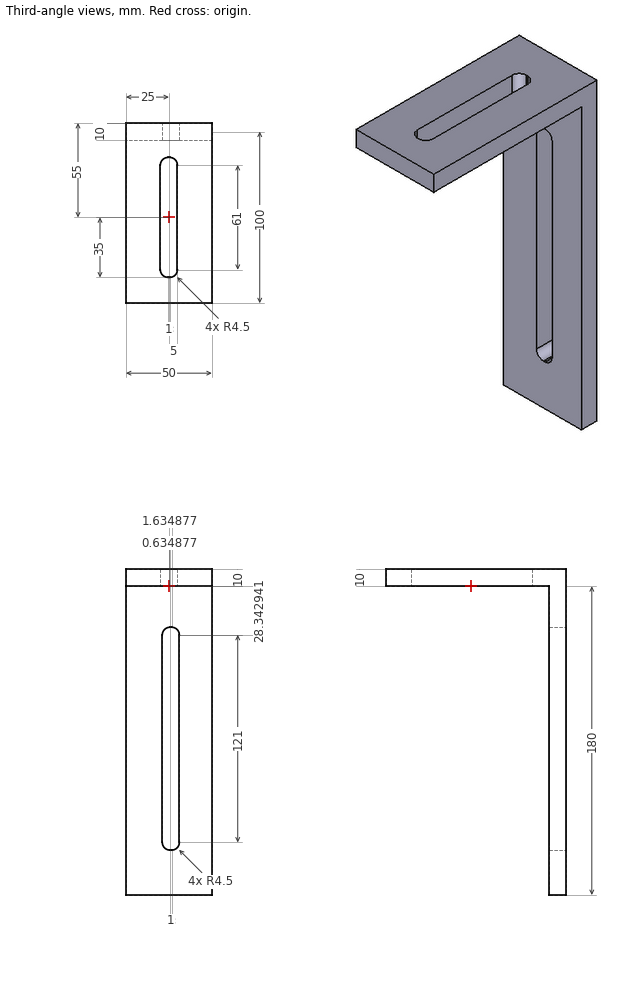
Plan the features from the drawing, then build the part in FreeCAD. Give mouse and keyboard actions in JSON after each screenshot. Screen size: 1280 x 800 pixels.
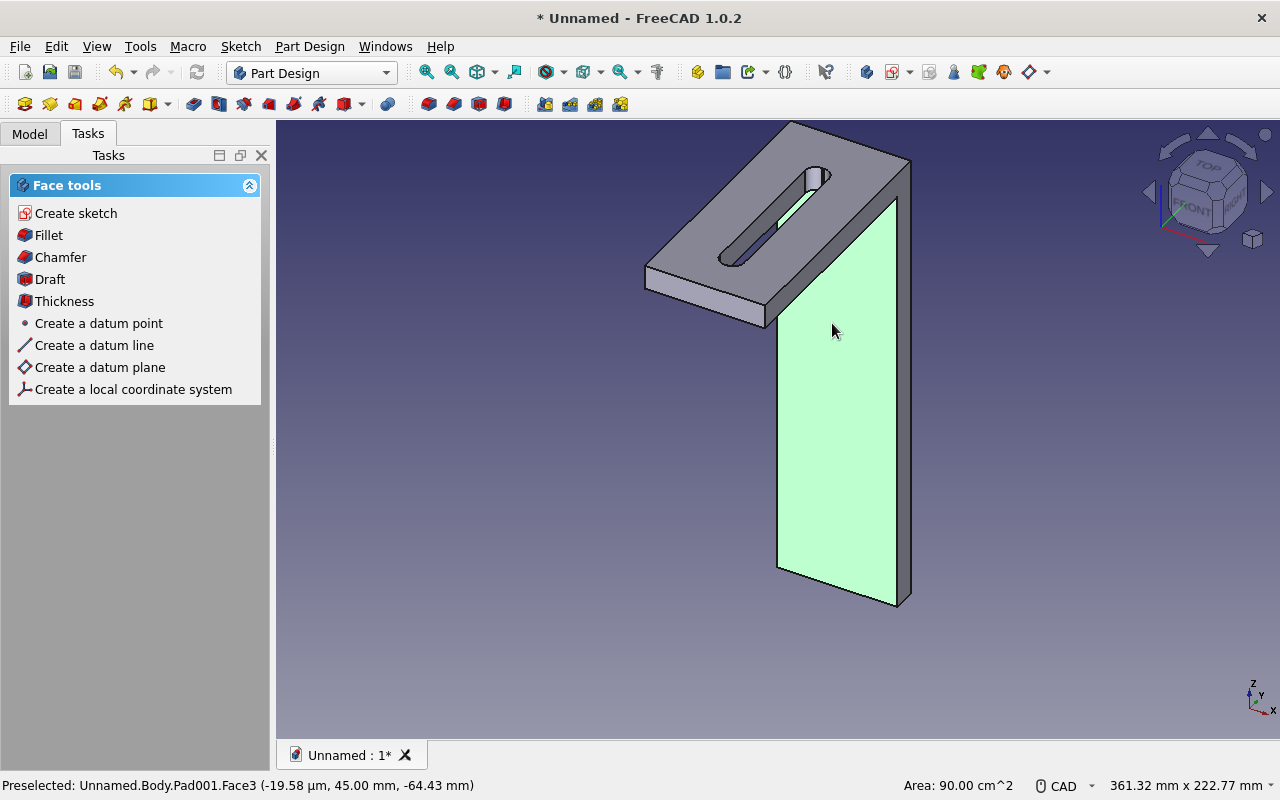
{"action": "left_click", "coordinate": [892, 72]}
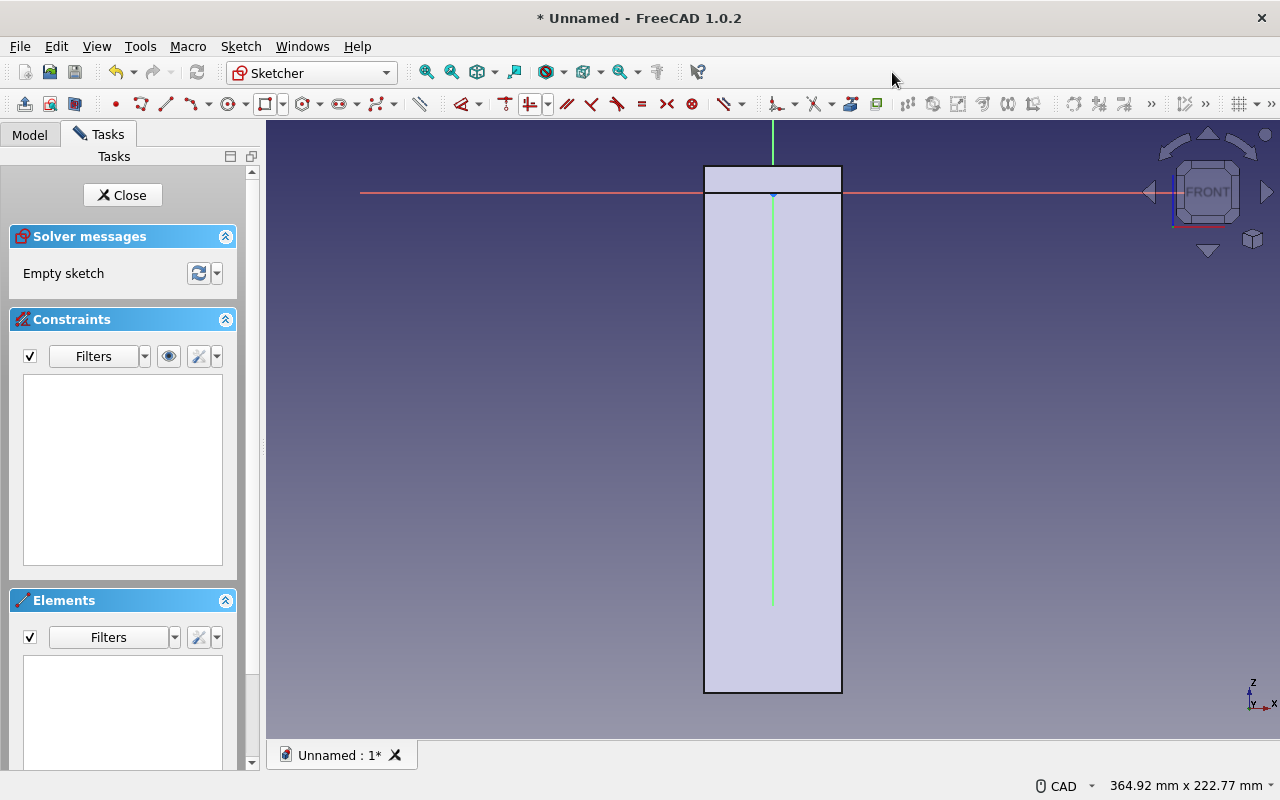
{"action": "left_click", "coordinate": [166, 104]}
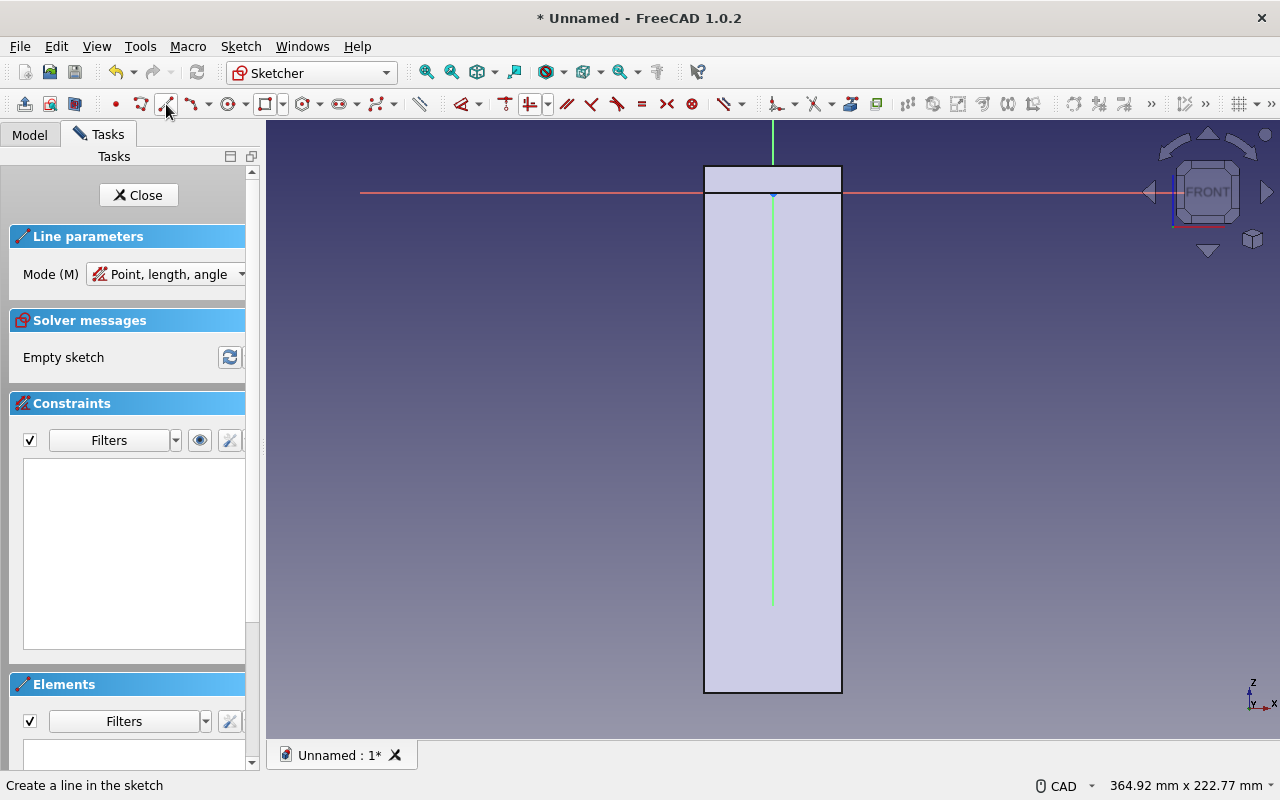
{"action": "scroll", "coordinate": [775, 621], "scroll_direction": "up", "scroll_amount": 11}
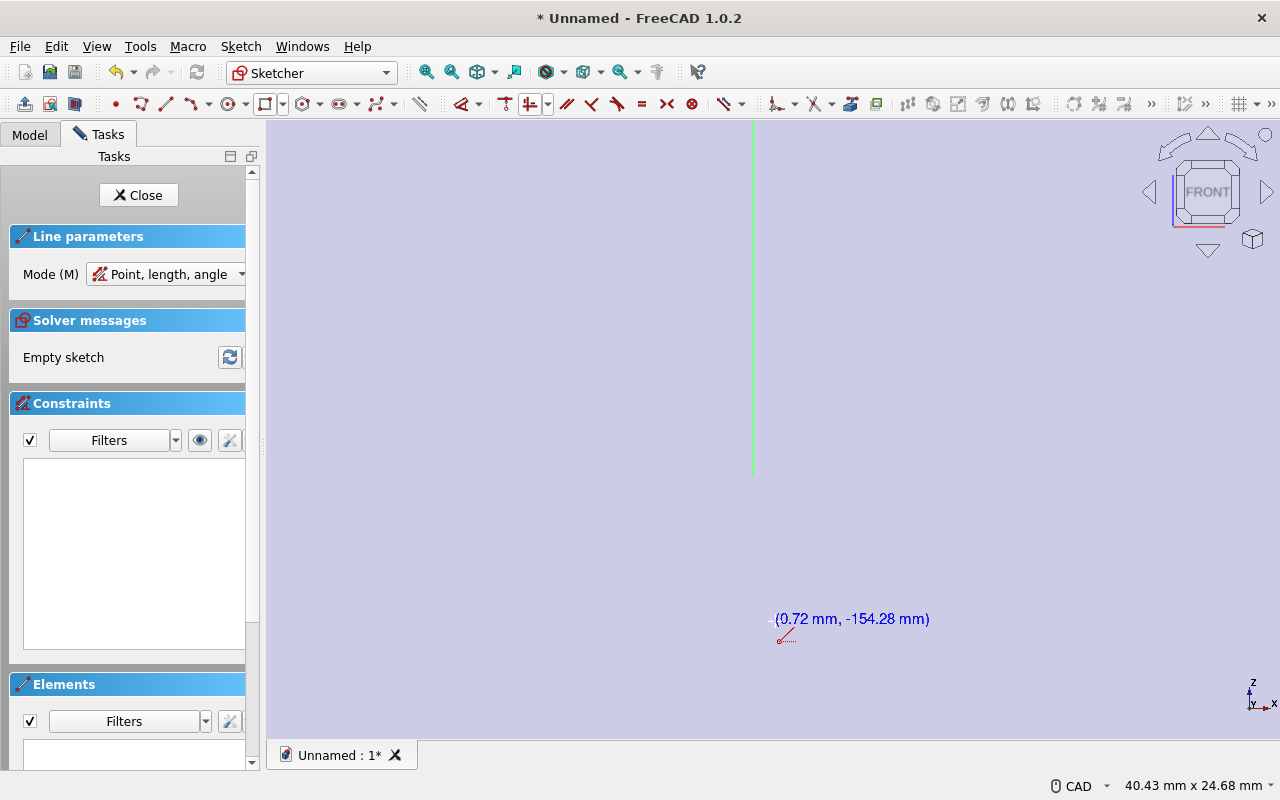
{"action": "left_click", "coordinate": [769, 613]}
{"action": "left_click", "coordinate": [794, 613]}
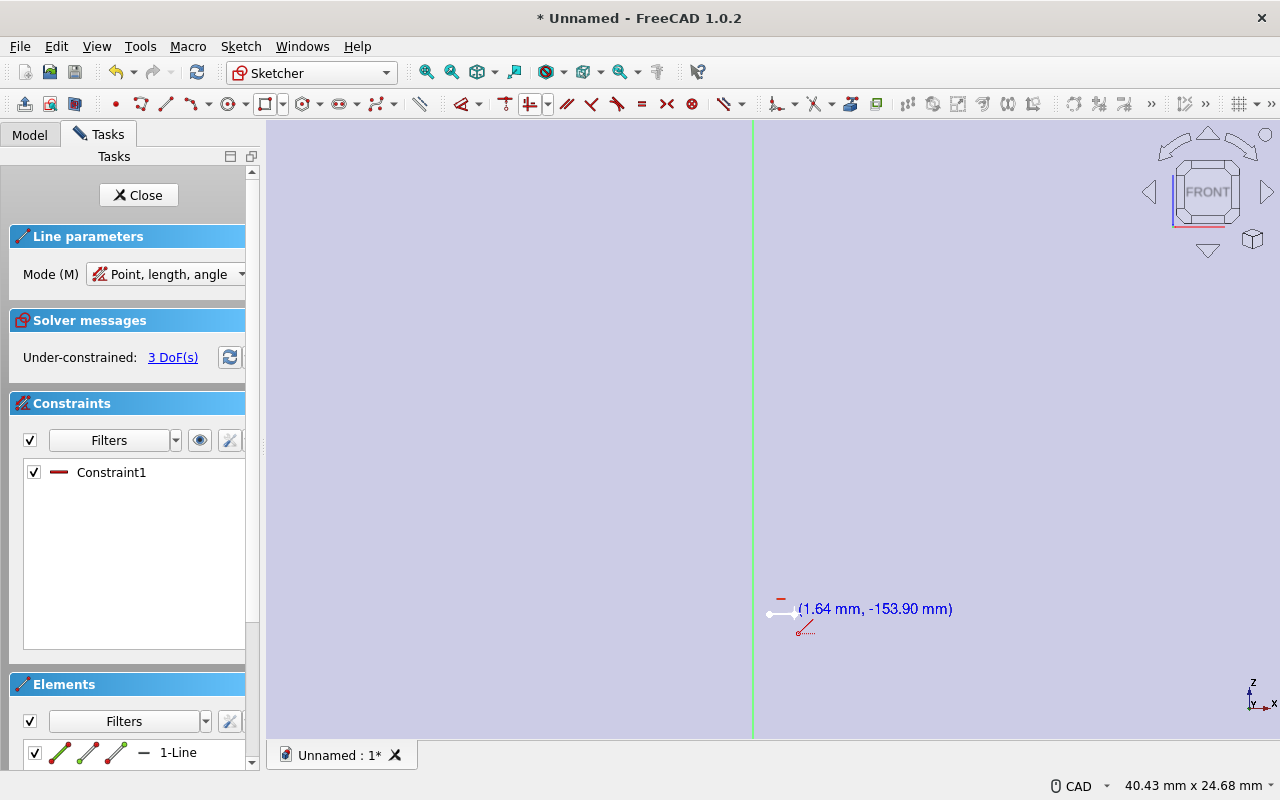
{"action": "scroll", "coordinate": [695, 647], "scroll_direction": "down", "scroll_amount": 11}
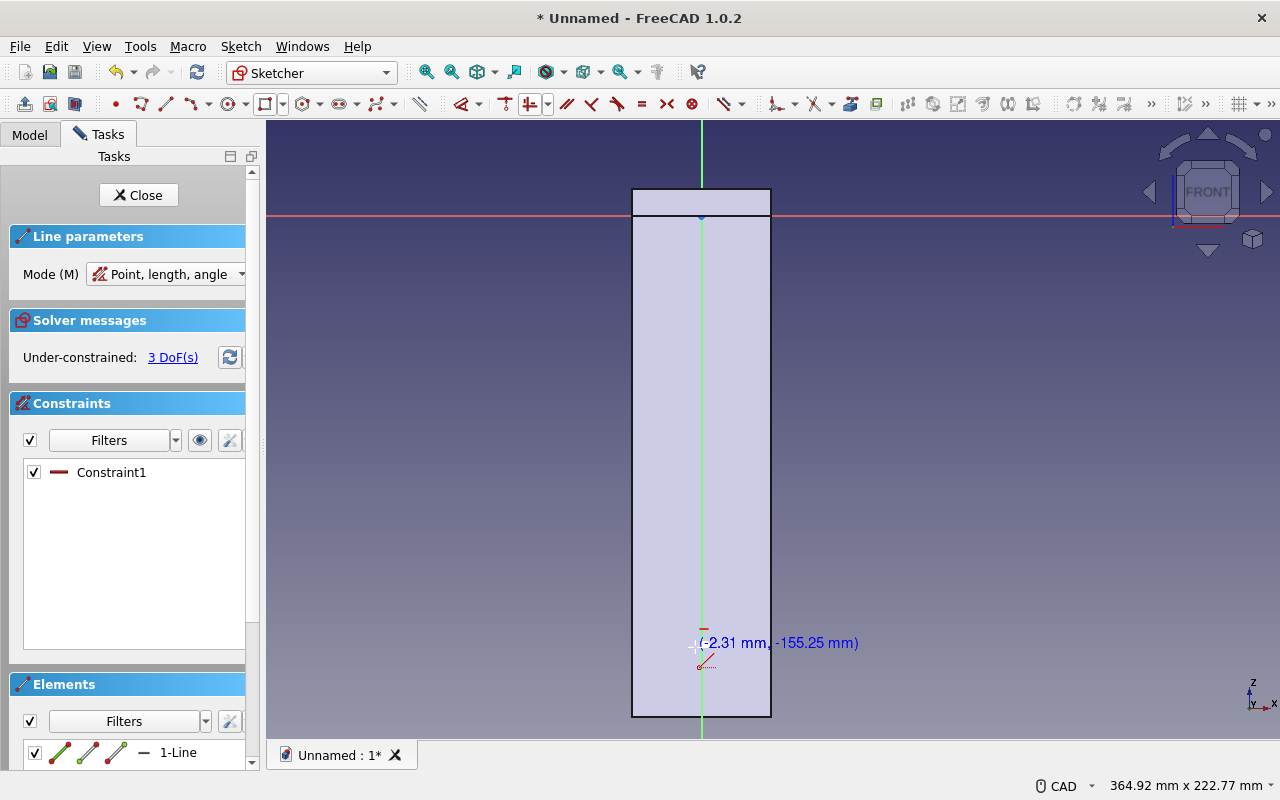
{"action": "left_click", "coordinate": [719, 631]}
{"action": "left_click", "coordinate": [719, 295]}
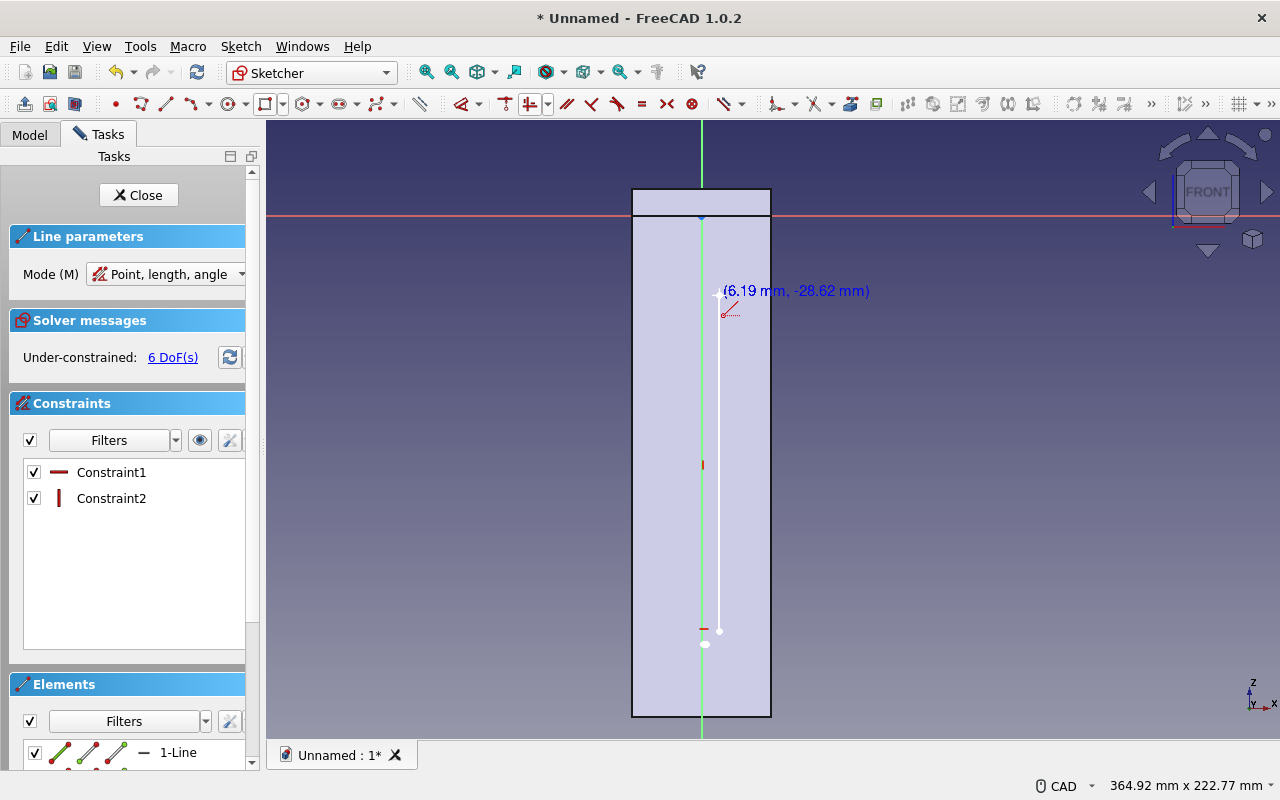
{"action": "scroll", "coordinate": [706, 283], "scroll_direction": "up", "scroll_amount": 7}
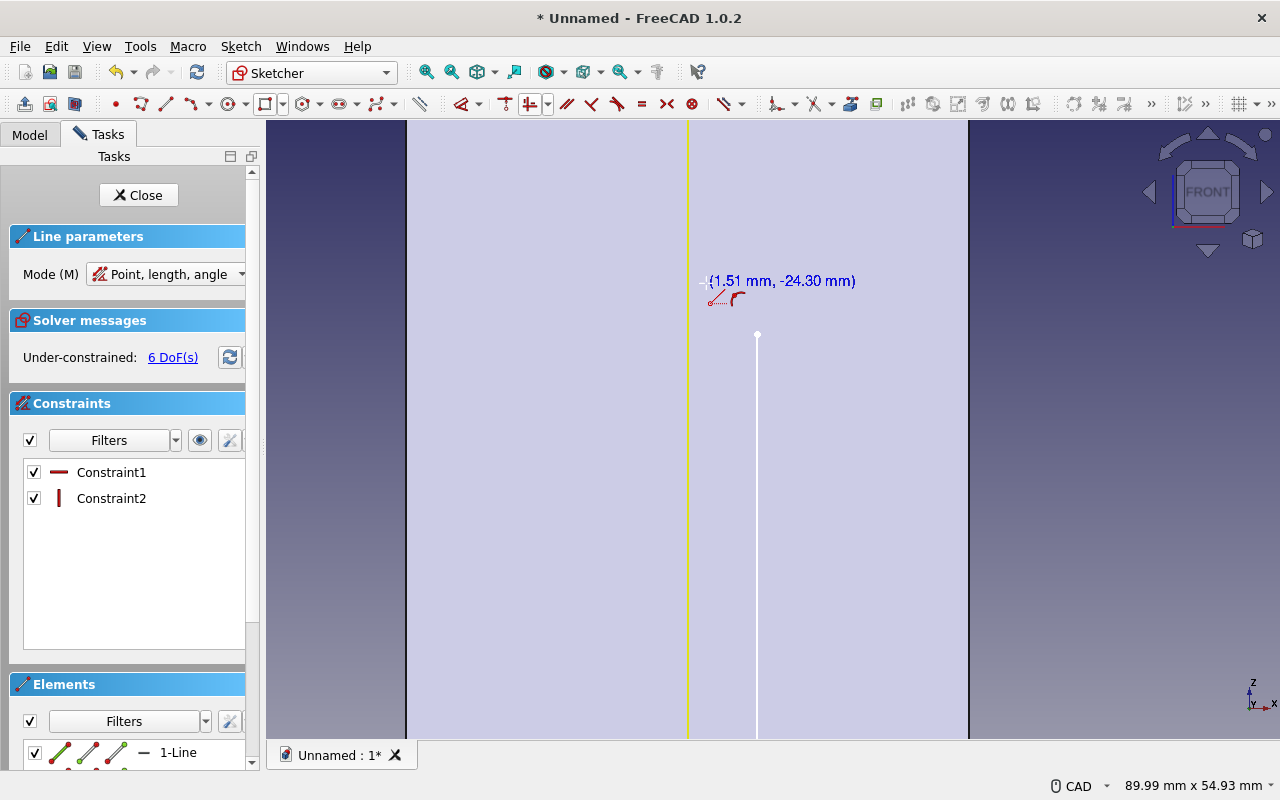
{"action": "left_click", "coordinate": [706, 281]}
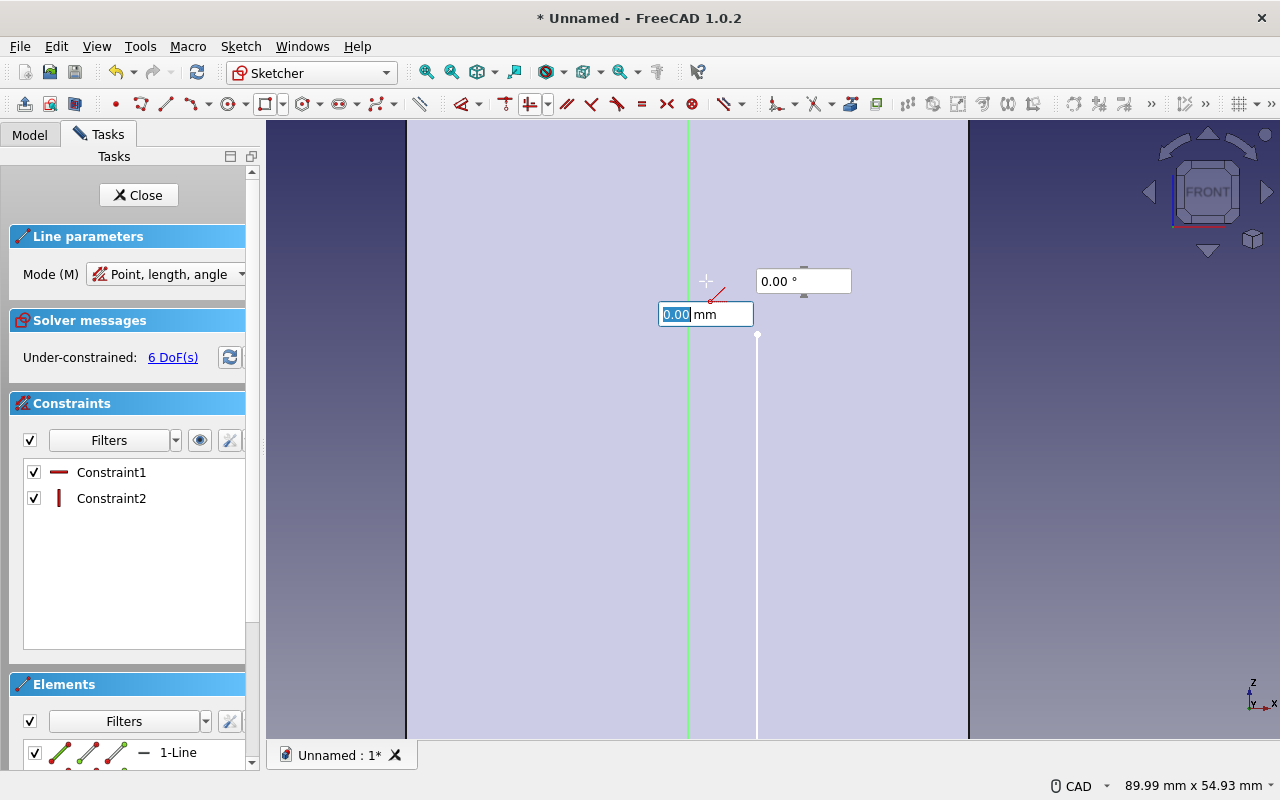
{"action": "scroll", "coordinate": [695, 281], "scroll_direction": "up", "scroll_amount": 4}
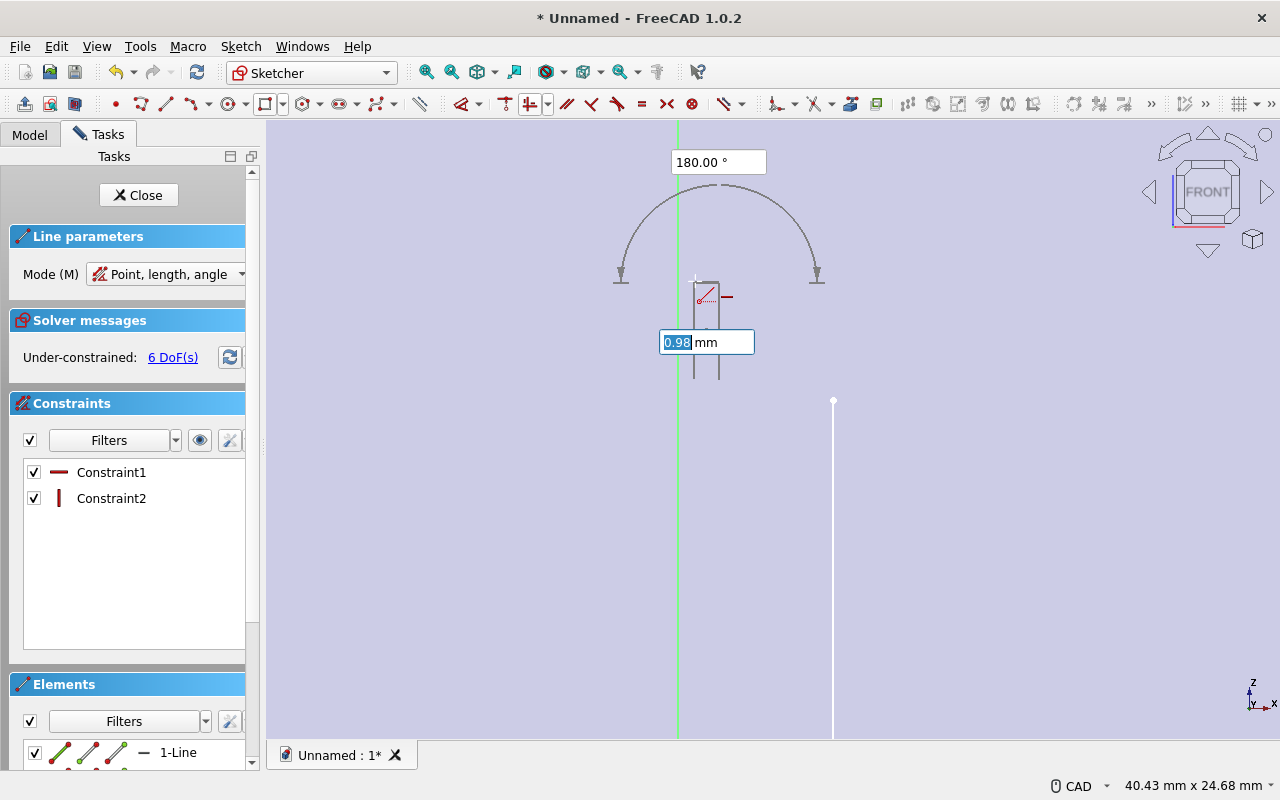
{"action": "left_click", "coordinate": [694, 281]}